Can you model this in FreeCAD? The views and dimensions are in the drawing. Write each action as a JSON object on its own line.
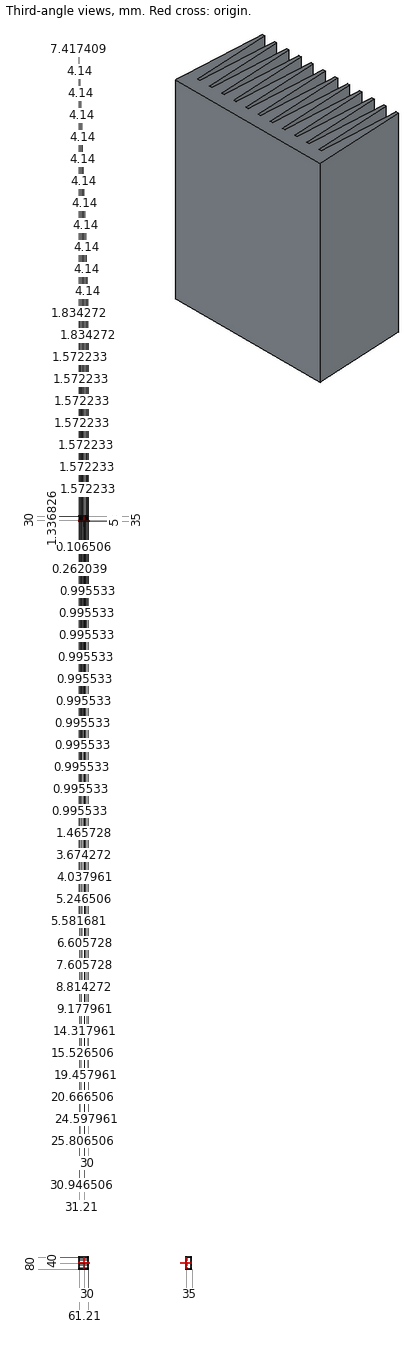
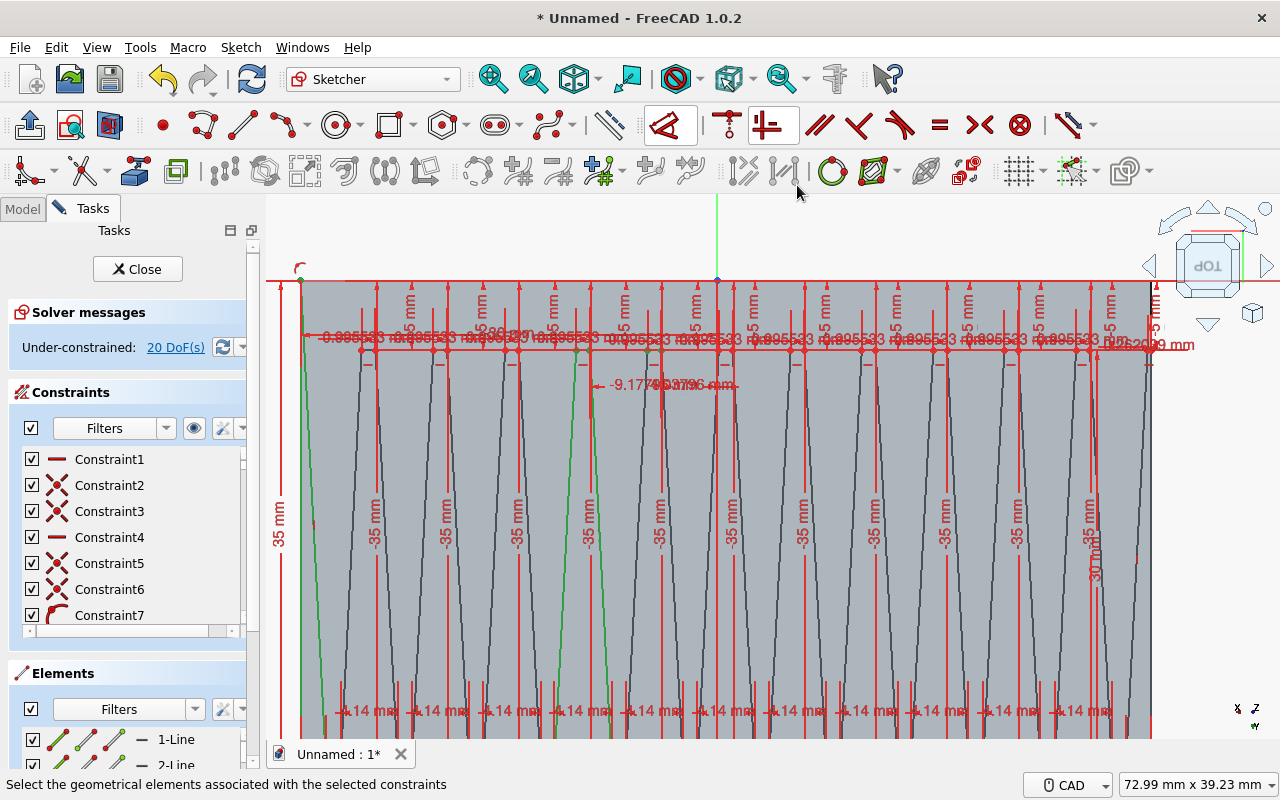
{"action": "scroll", "coordinate": [661, 349], "scroll_direction": "down", "scroll_amount": 2}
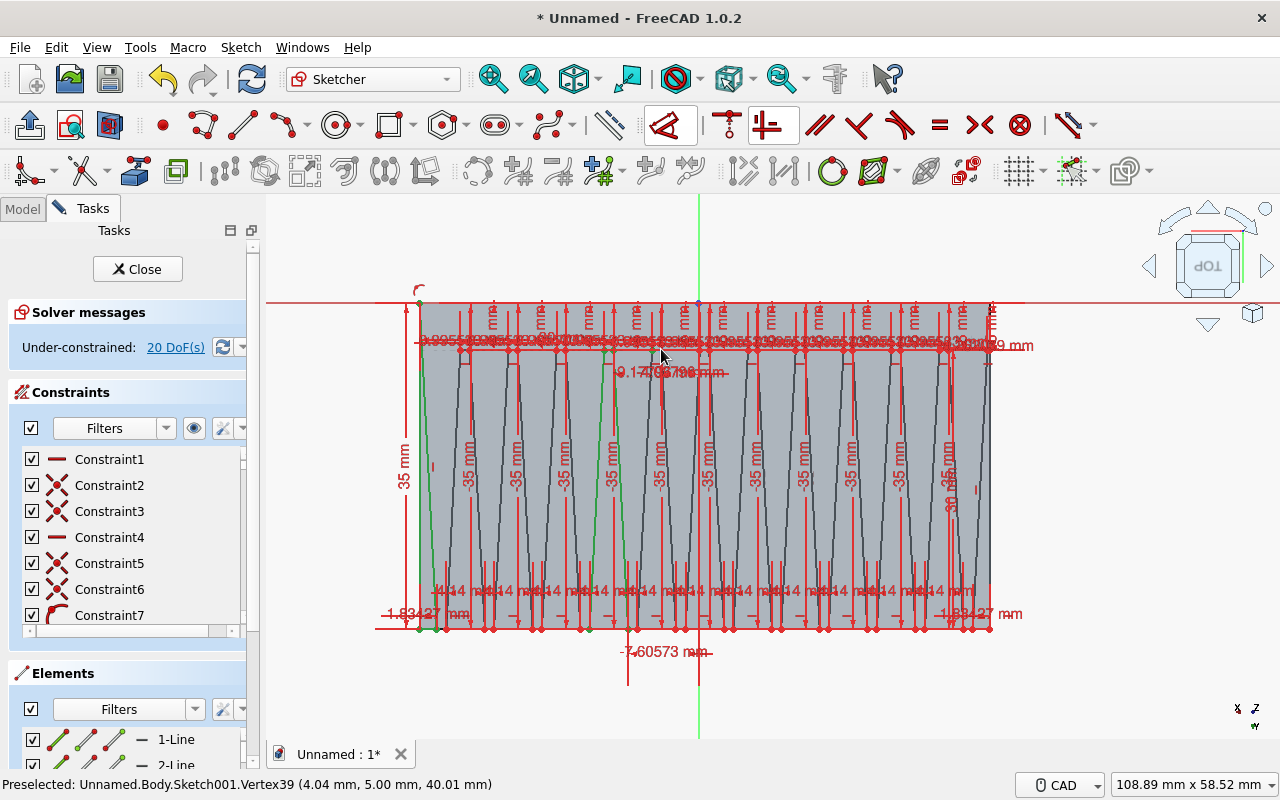
{"action": "scroll", "coordinate": [637, 629], "scroll_direction": "up", "scroll_amount": 2}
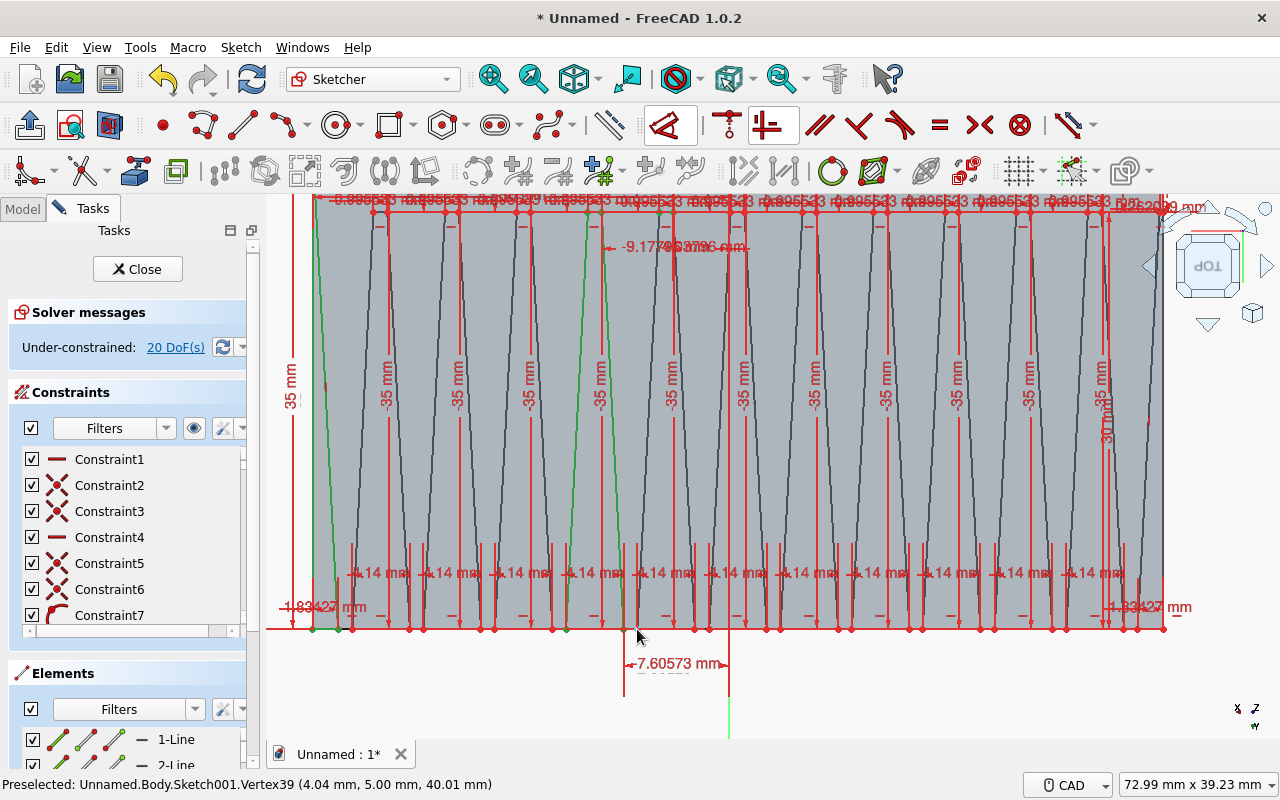
{"action": "left_click", "coordinate": [637, 629]}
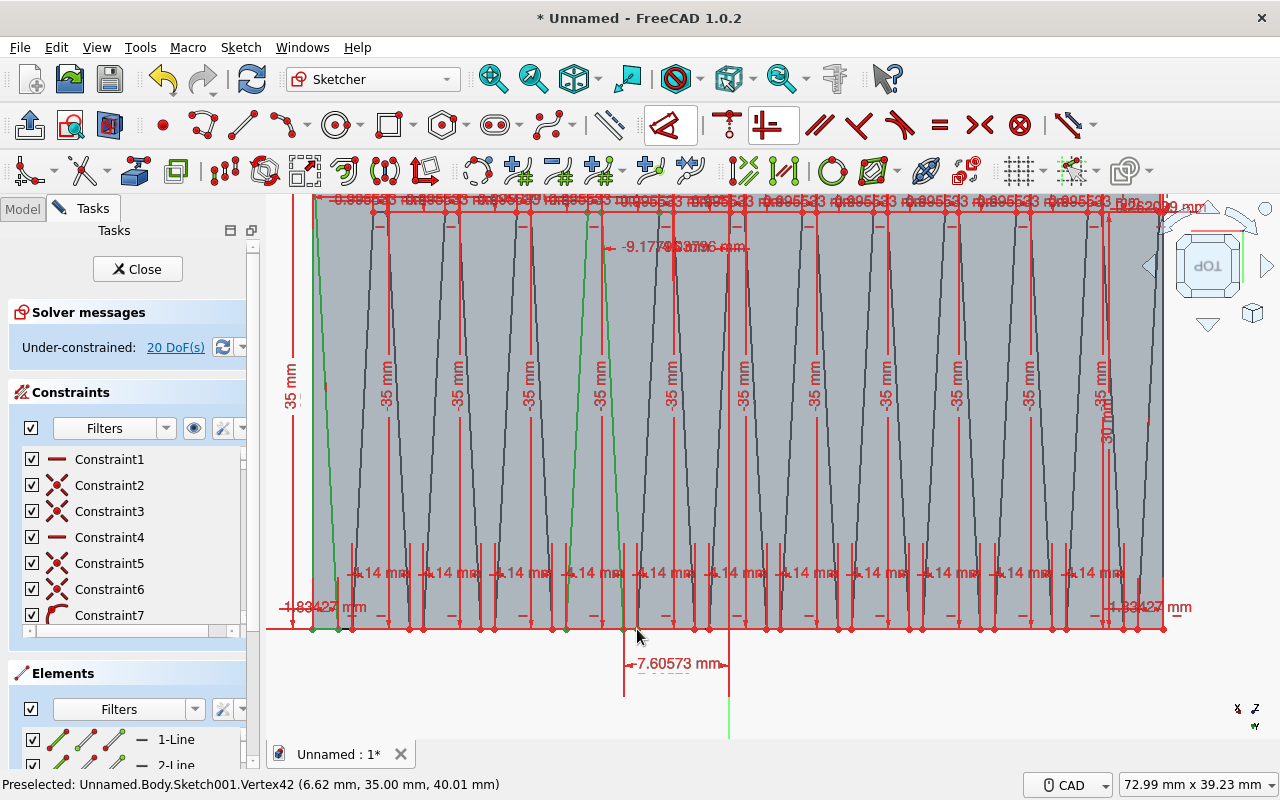
{"action": "key", "text": "l"}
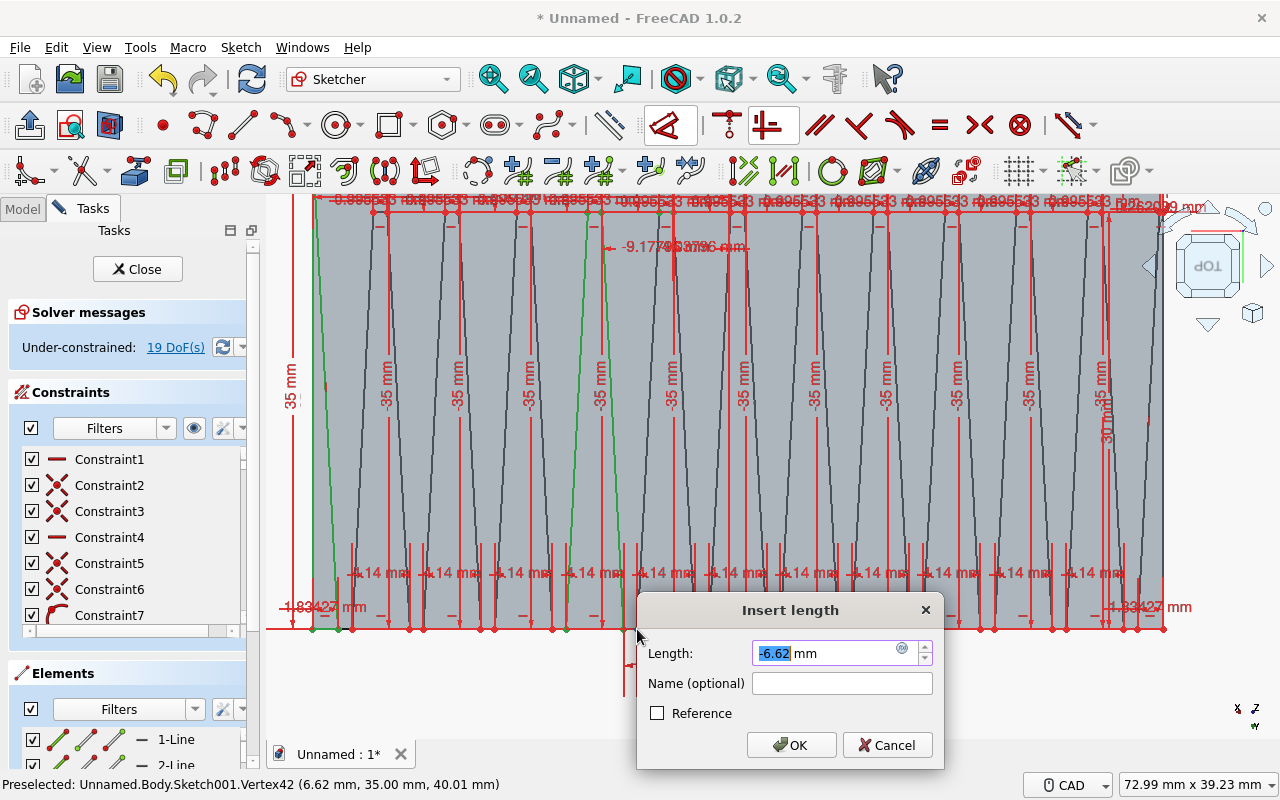
{"action": "type", "text": "-6.605728"}
{"action": "key", "text": "Return"}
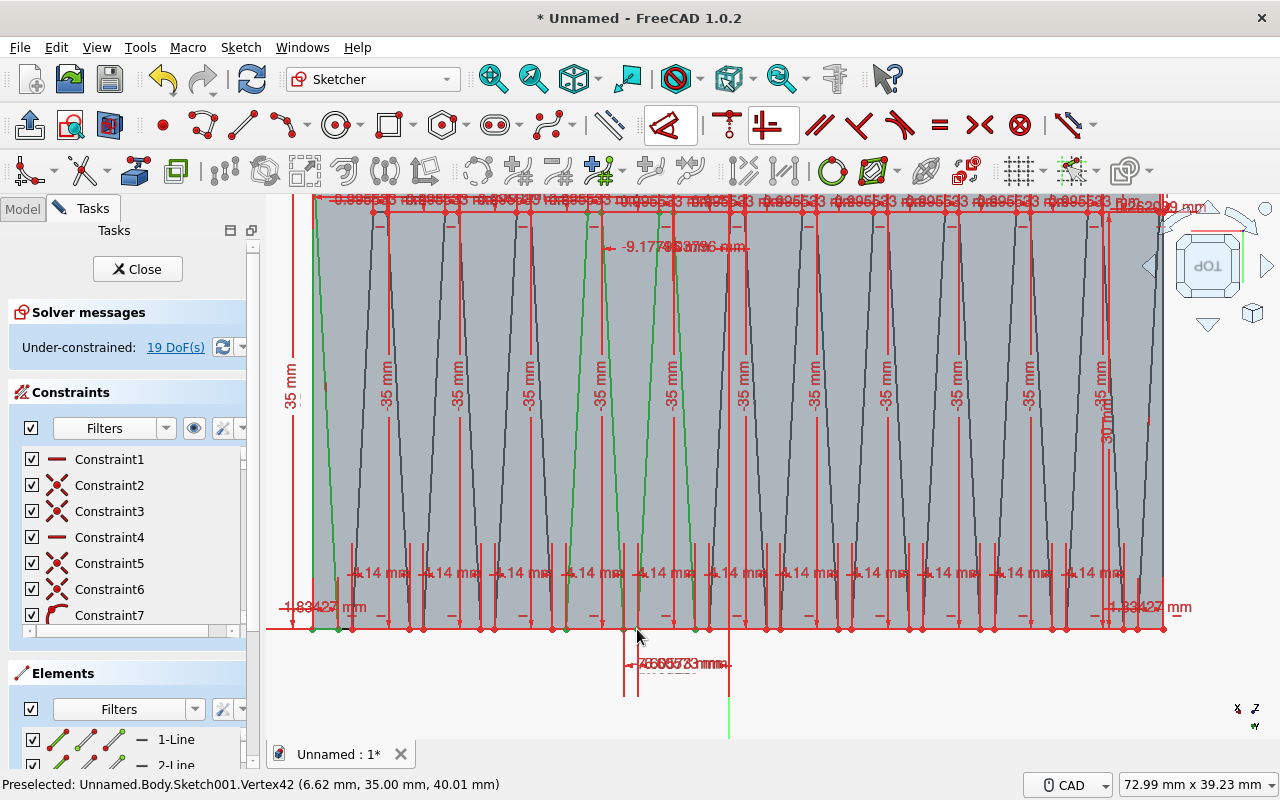
{"action": "scroll", "coordinate": [637, 630], "scroll_direction": "down", "scroll_amount": 2}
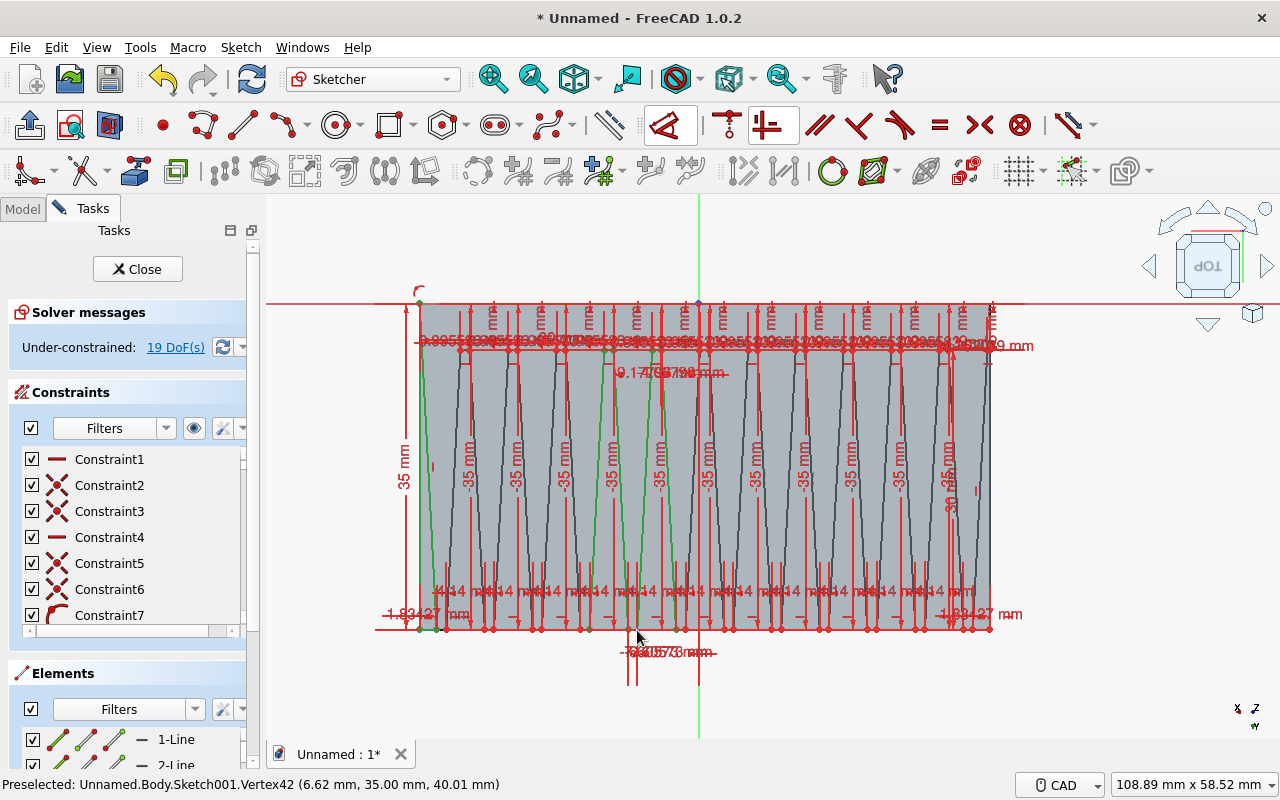
{"action": "scroll", "coordinate": [700, 350], "scroll_direction": "up", "scroll_amount": 19}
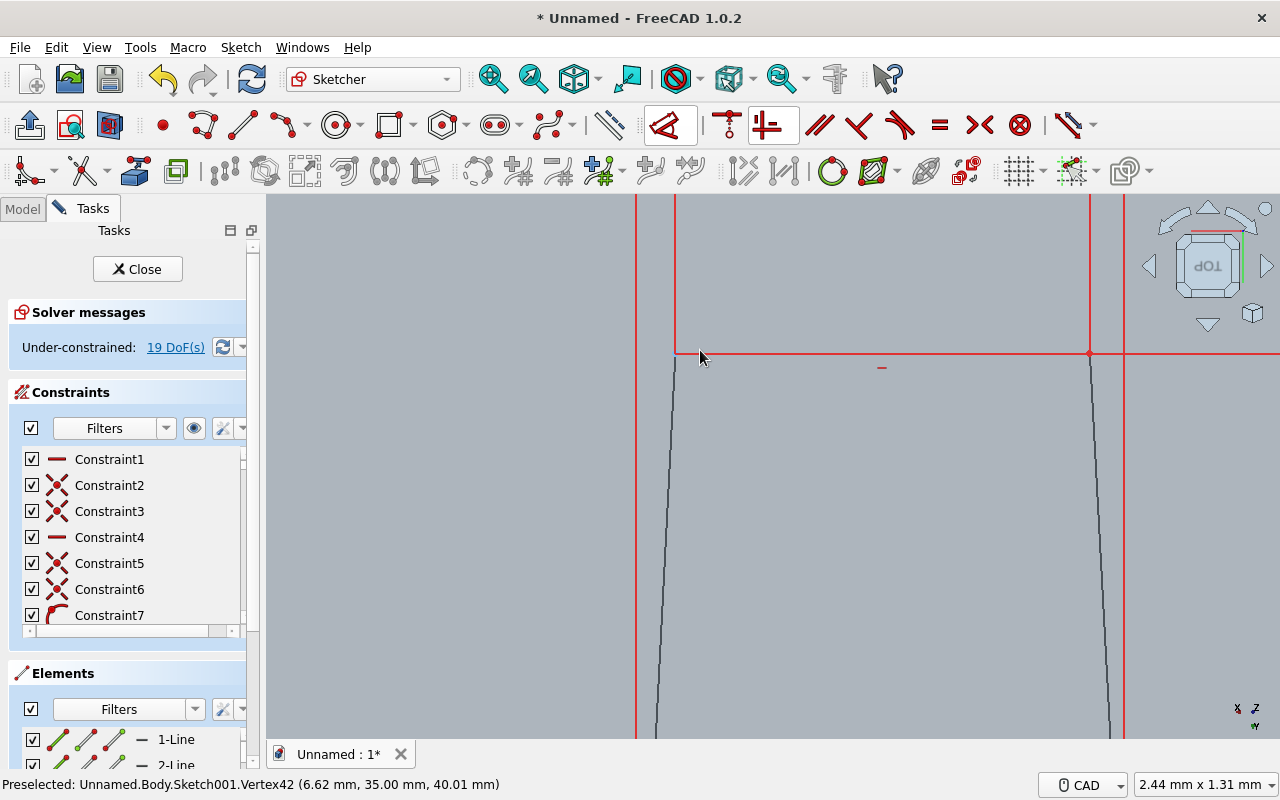
{"action": "left_click", "coordinate": [675, 354]}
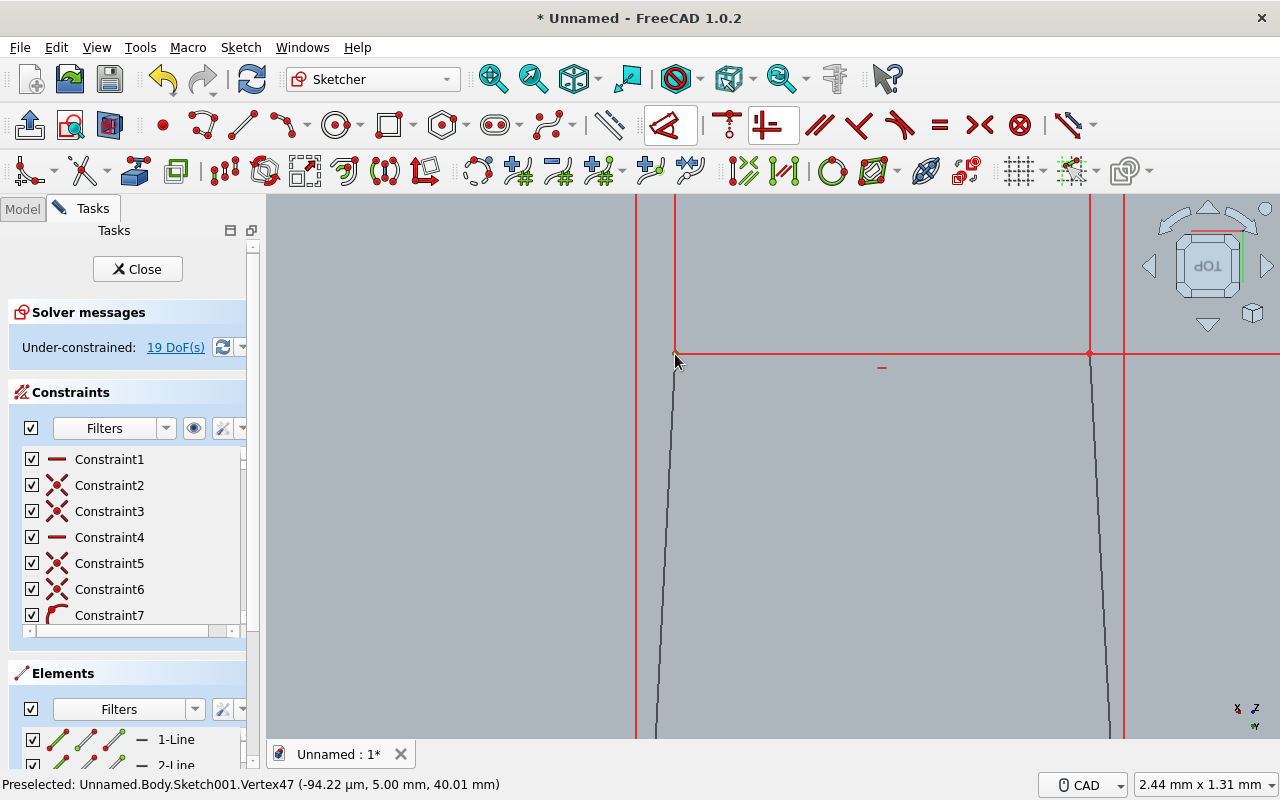
{"action": "left_click", "coordinate": [692, 126]}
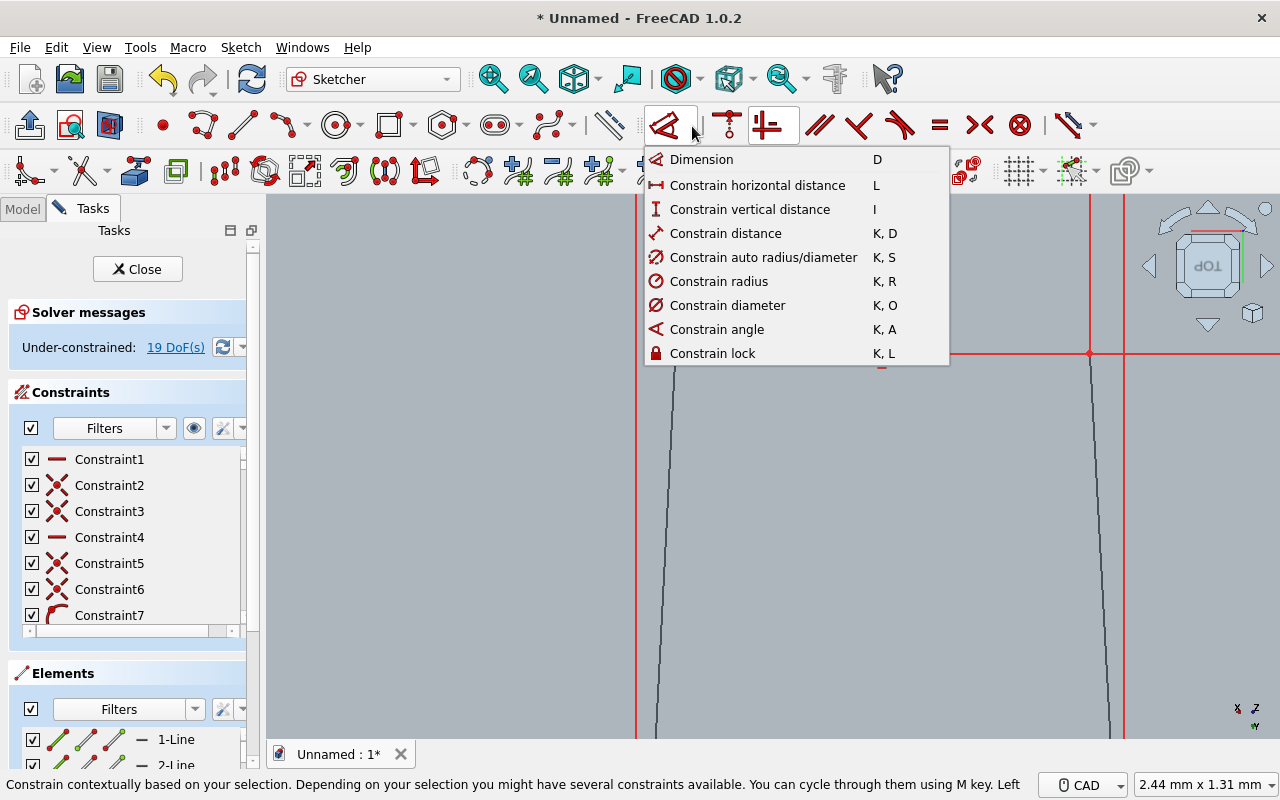
{"action": "left_click", "coordinate": [797, 185]}